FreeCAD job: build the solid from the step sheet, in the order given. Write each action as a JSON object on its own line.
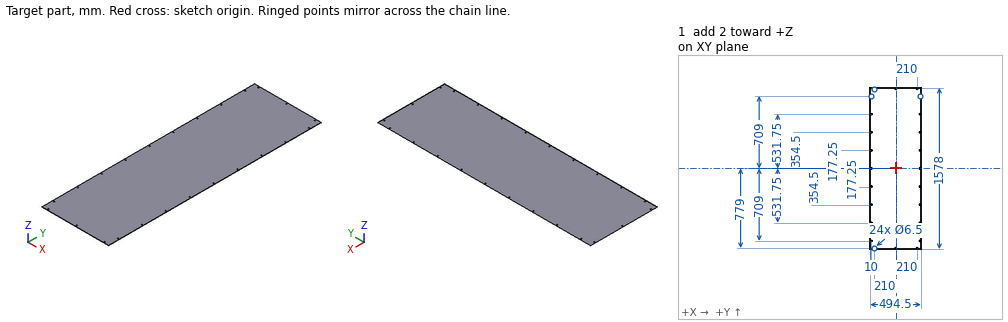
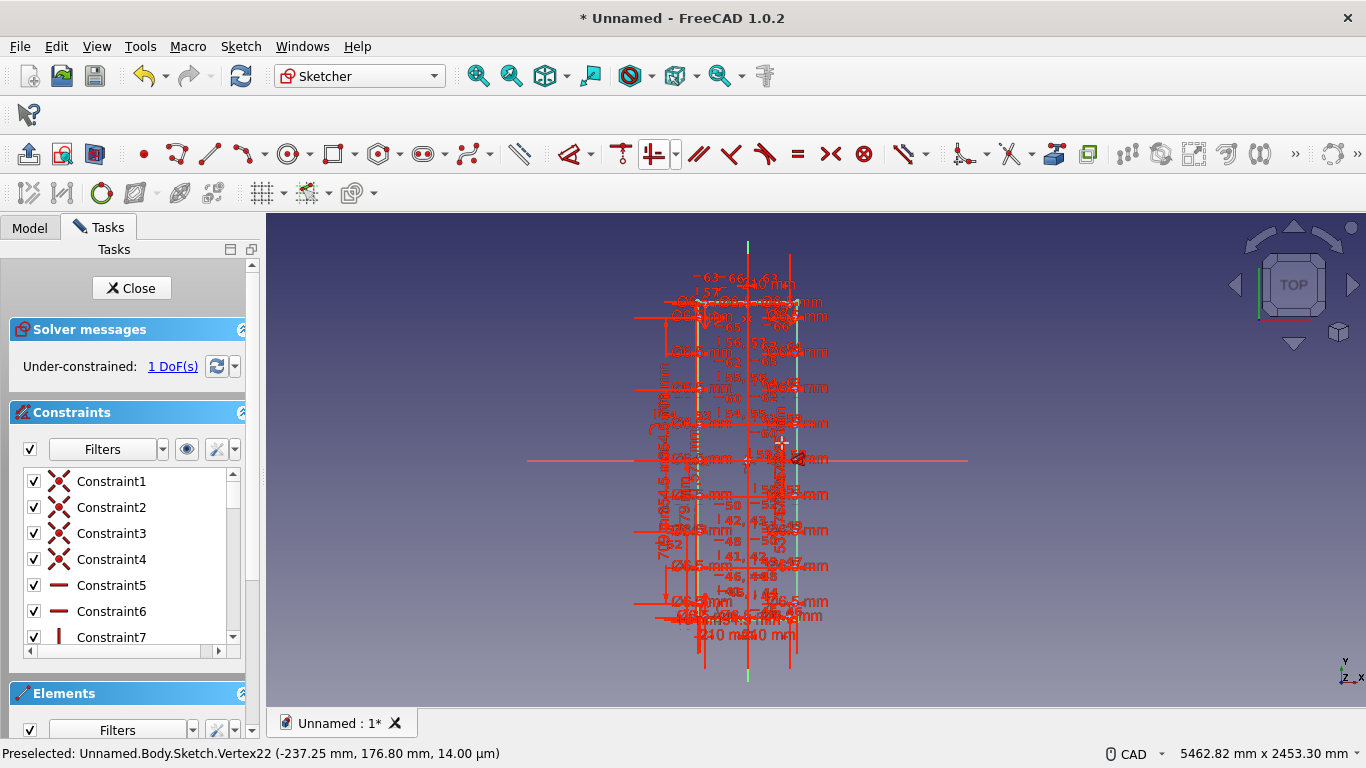
{"action": "left_click", "coordinate": [700, 354]}
{"action": "left_click", "coordinate": [782, 407]}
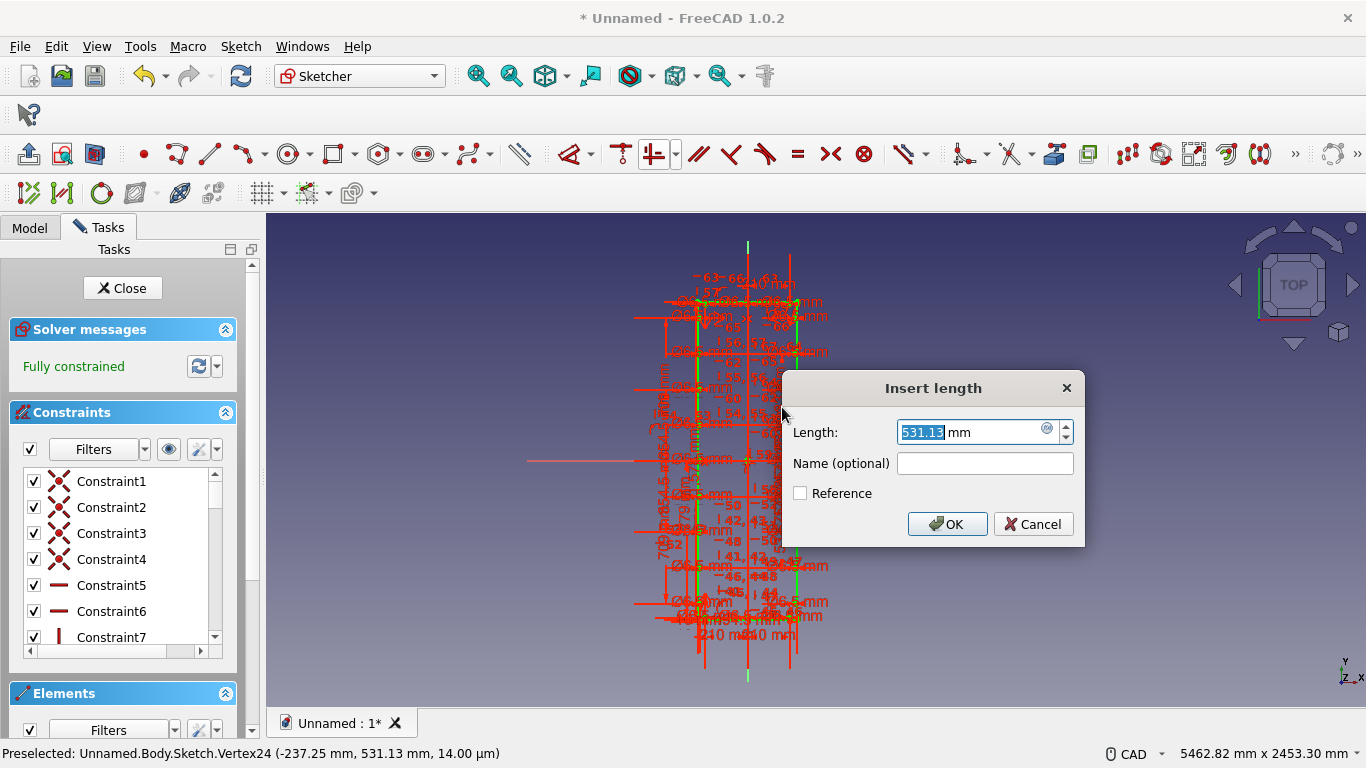
{"action": "type", "text": "531.75"}
{"action": "key", "text": "Return"}
{"action": "key", "text": "Escape"}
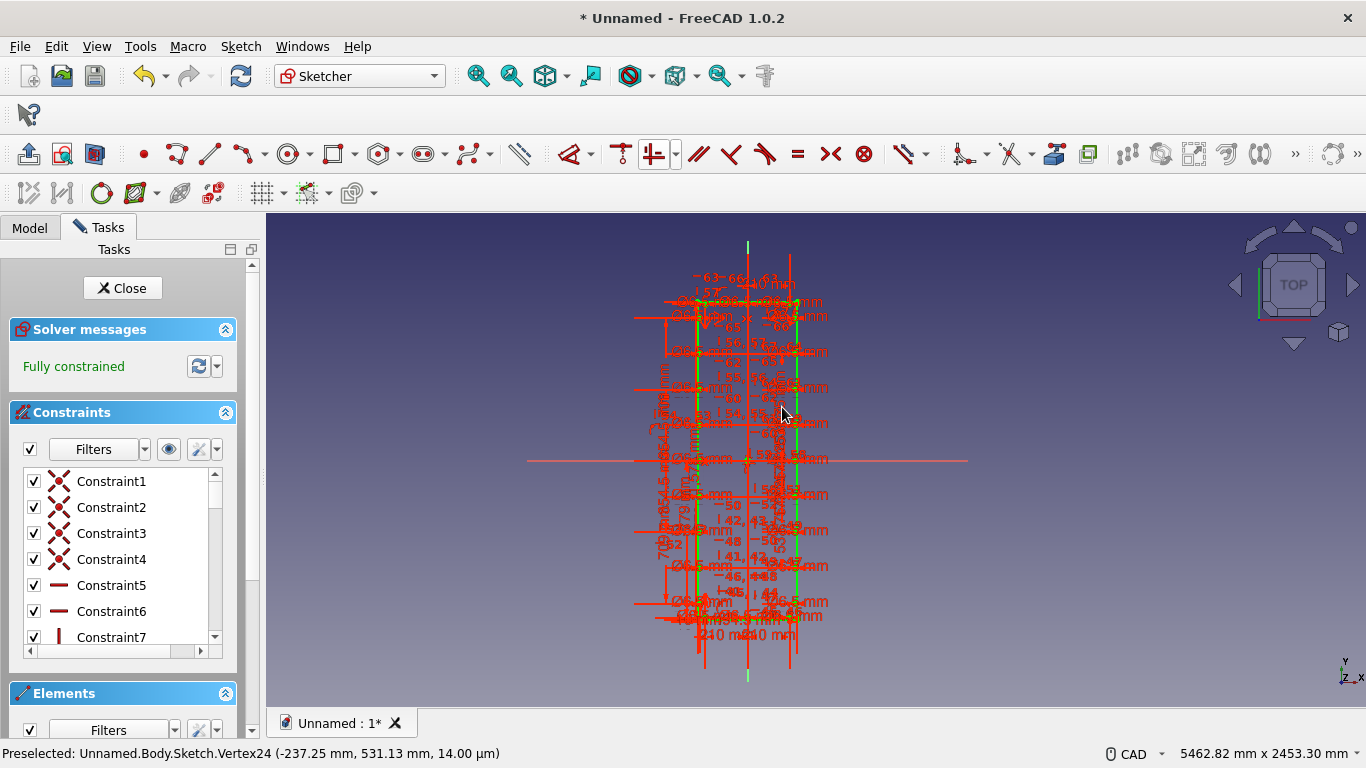
{"action": "left_click", "coordinate": [123, 288]}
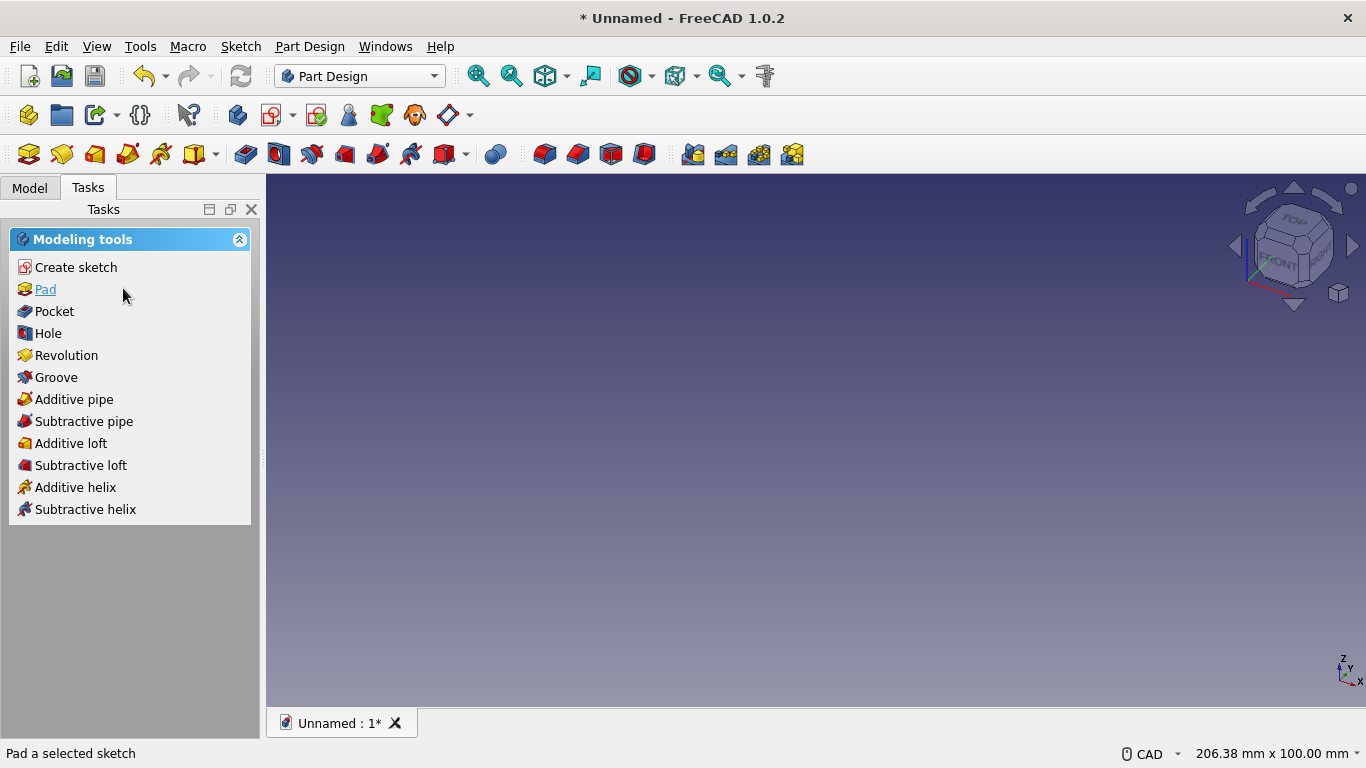
{"action": "left_click", "coordinate": [29, 154]}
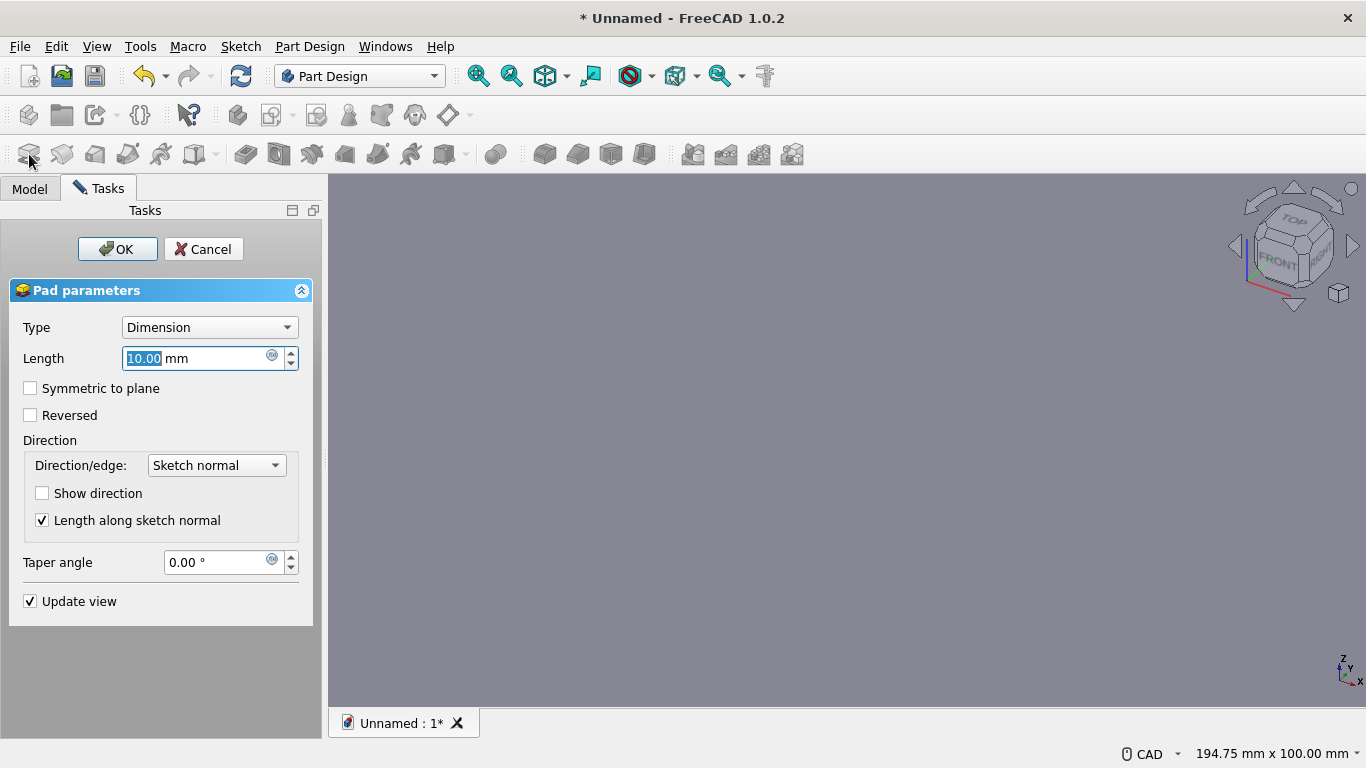
{"action": "type", "text": "2"}
{"action": "key", "text": "Tab"}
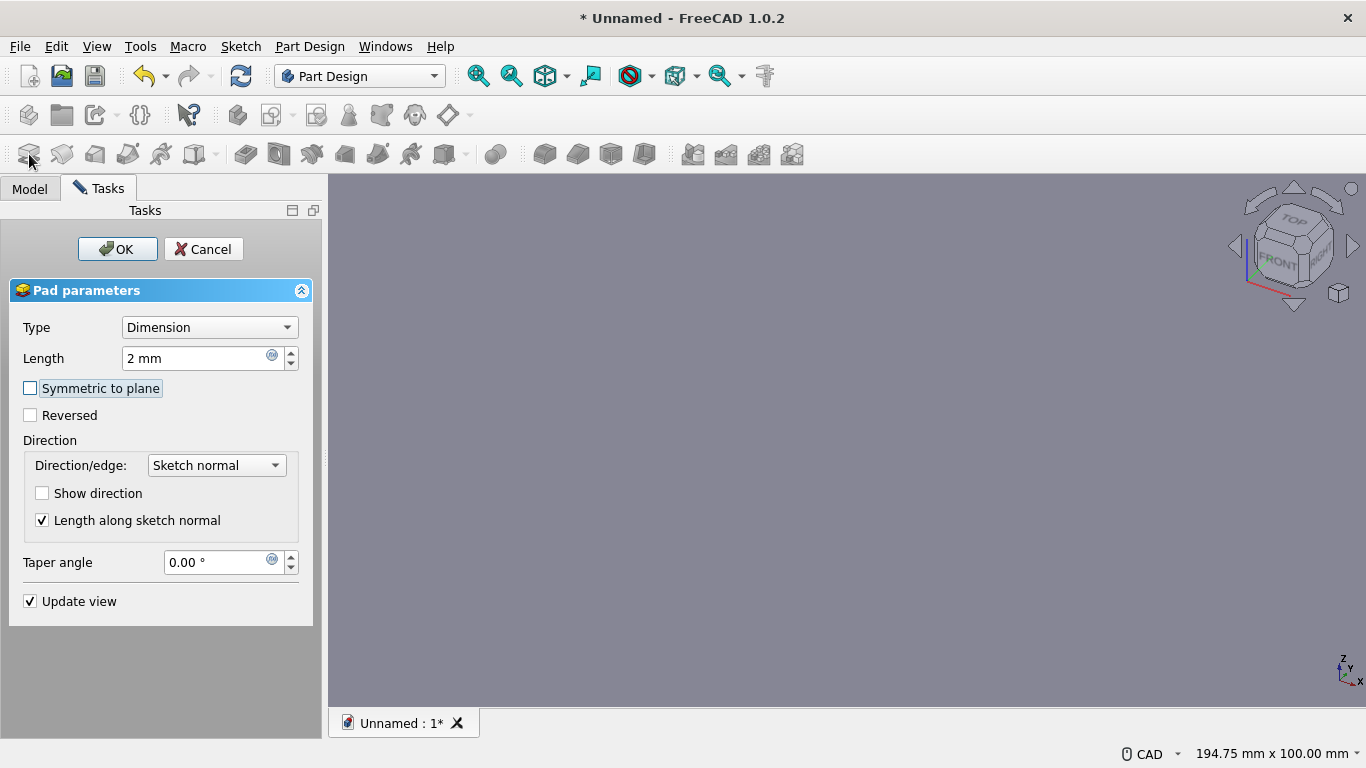
{"action": "left_click", "coordinate": [118, 249]}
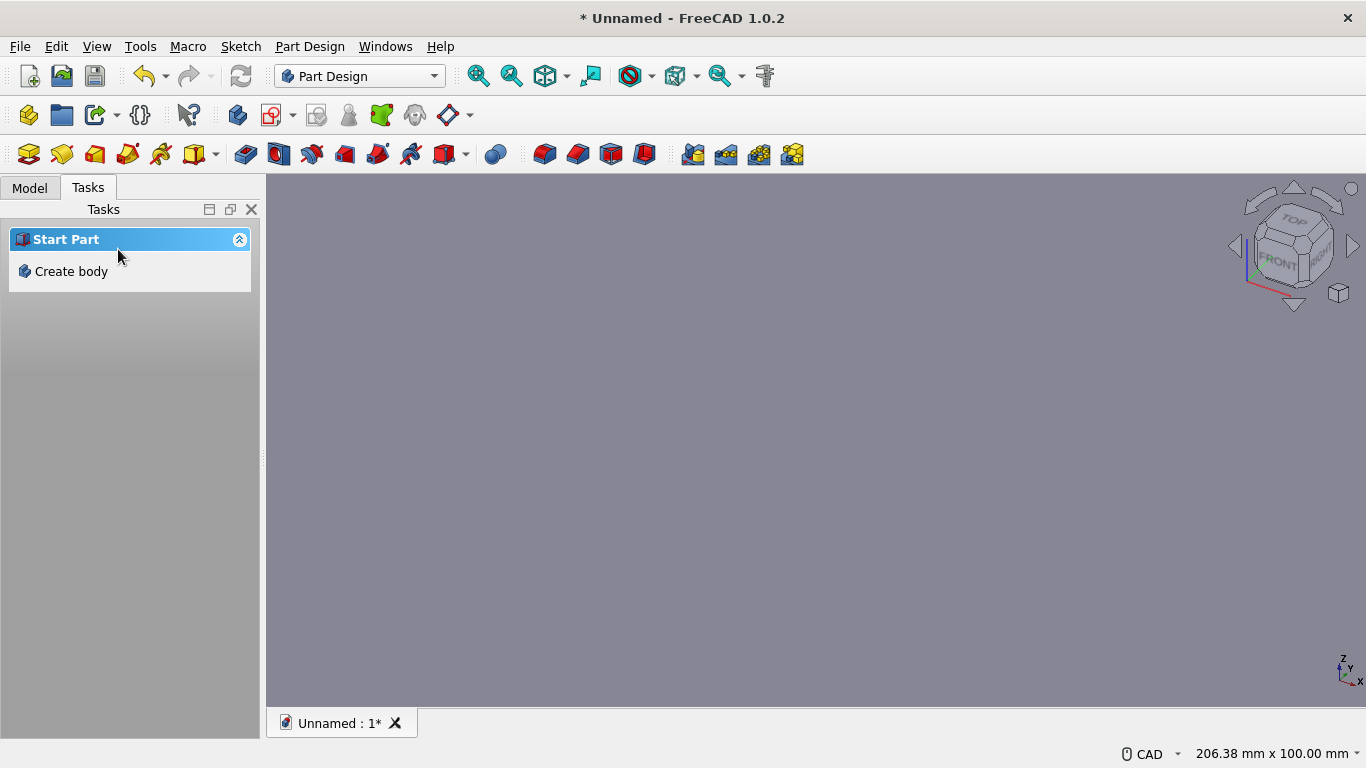
{"action": "key", "text": "0"}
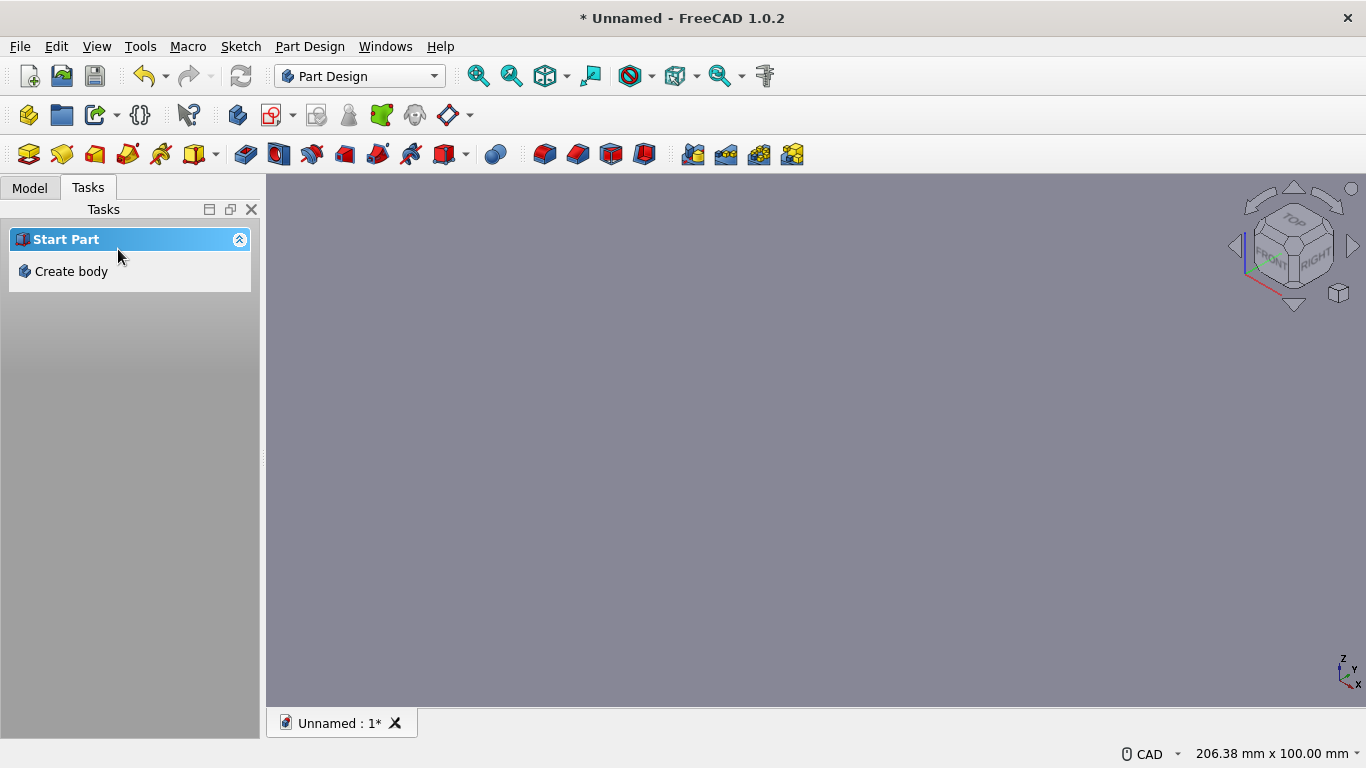
{"action": "key", "text": "v f"}